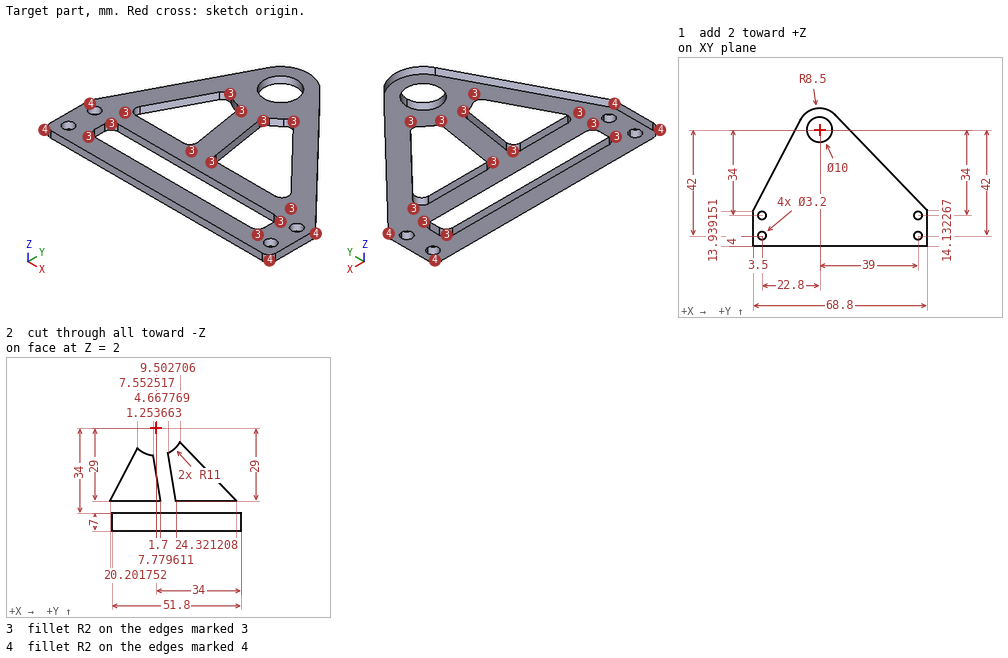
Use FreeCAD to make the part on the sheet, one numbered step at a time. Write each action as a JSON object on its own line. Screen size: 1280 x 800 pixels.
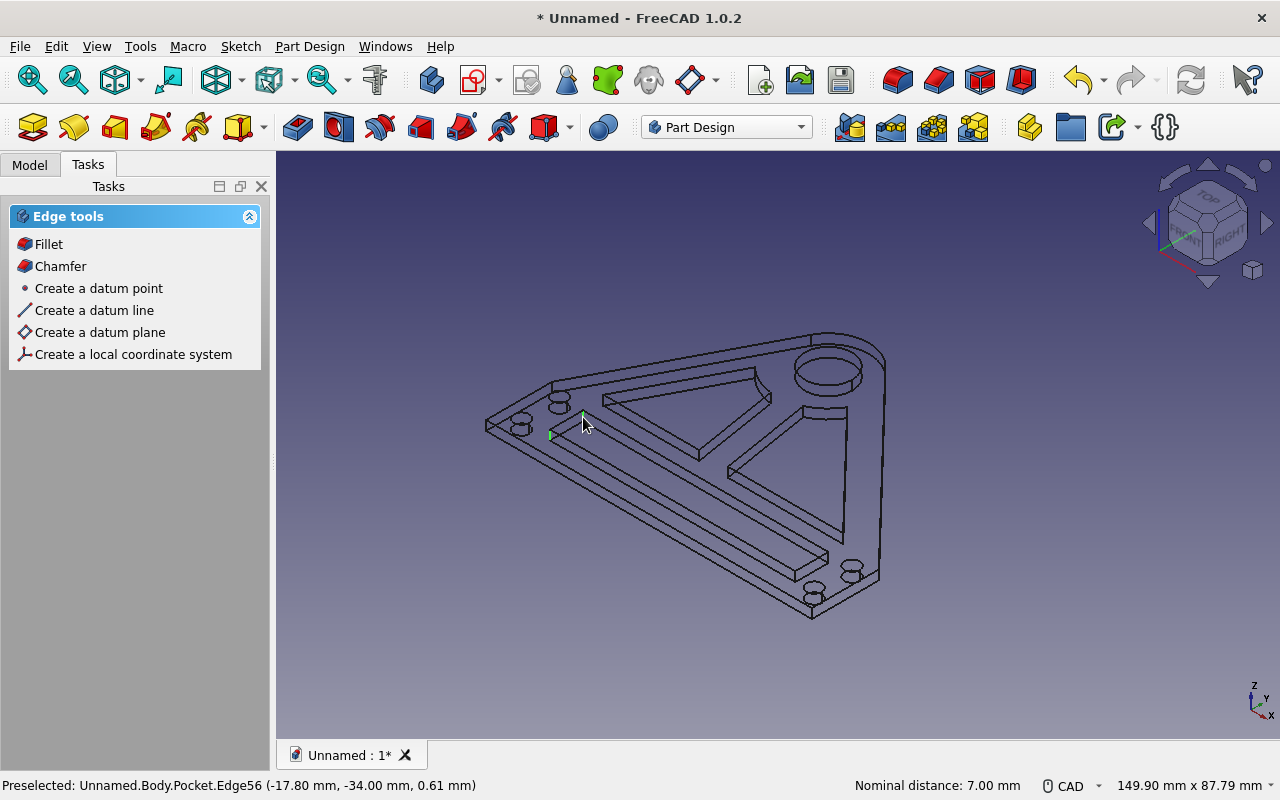
{"action": "left_click", "coordinate": [828, 559], "text": "ctrl"}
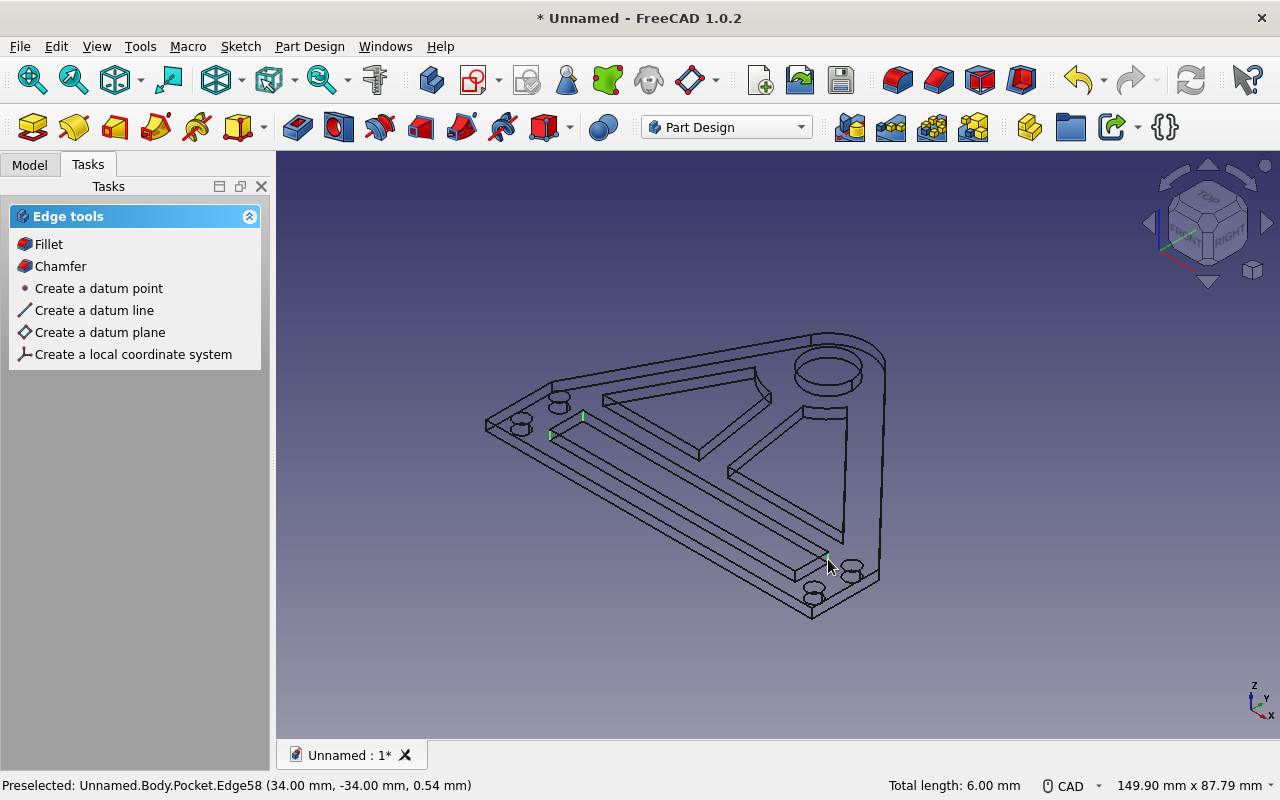
{"action": "left_click", "coordinate": [795, 577], "text": "ctrl"}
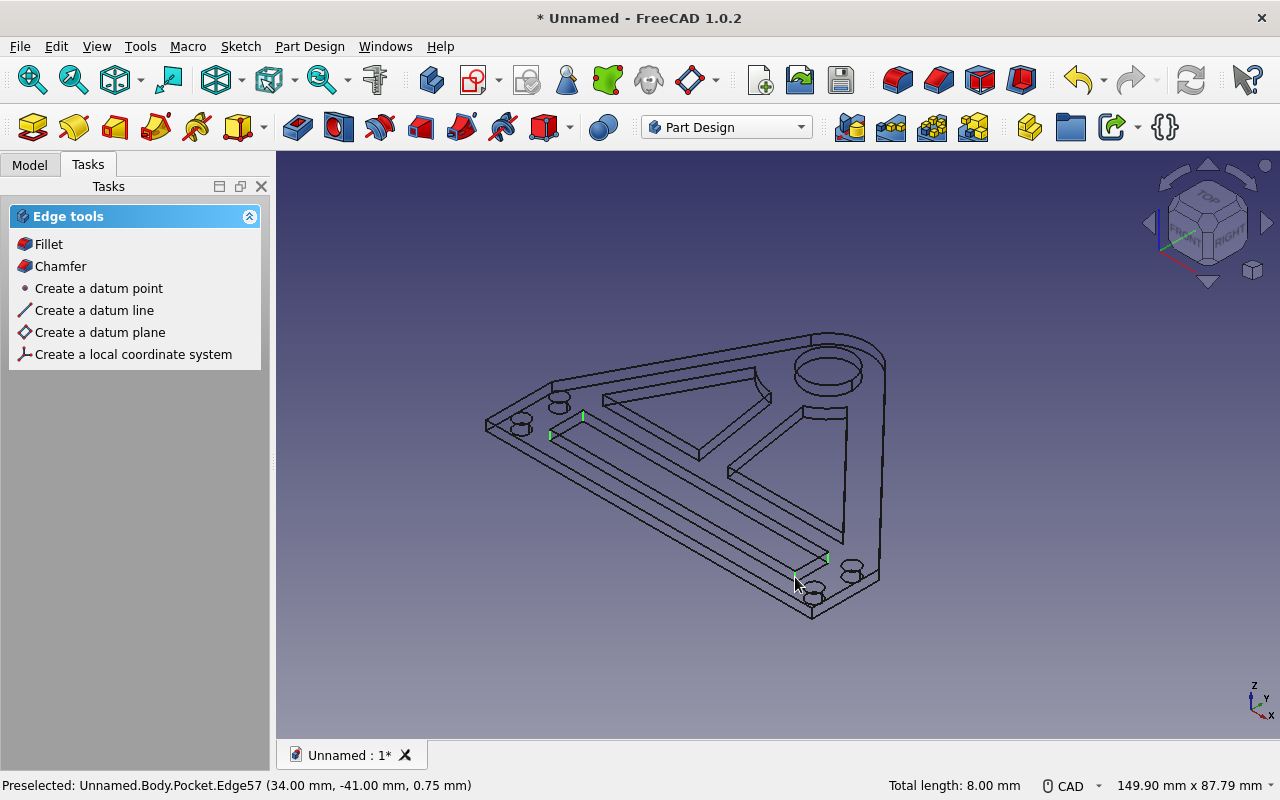
{"action": "left_click", "coordinate": [843, 539], "text": "ctrl"}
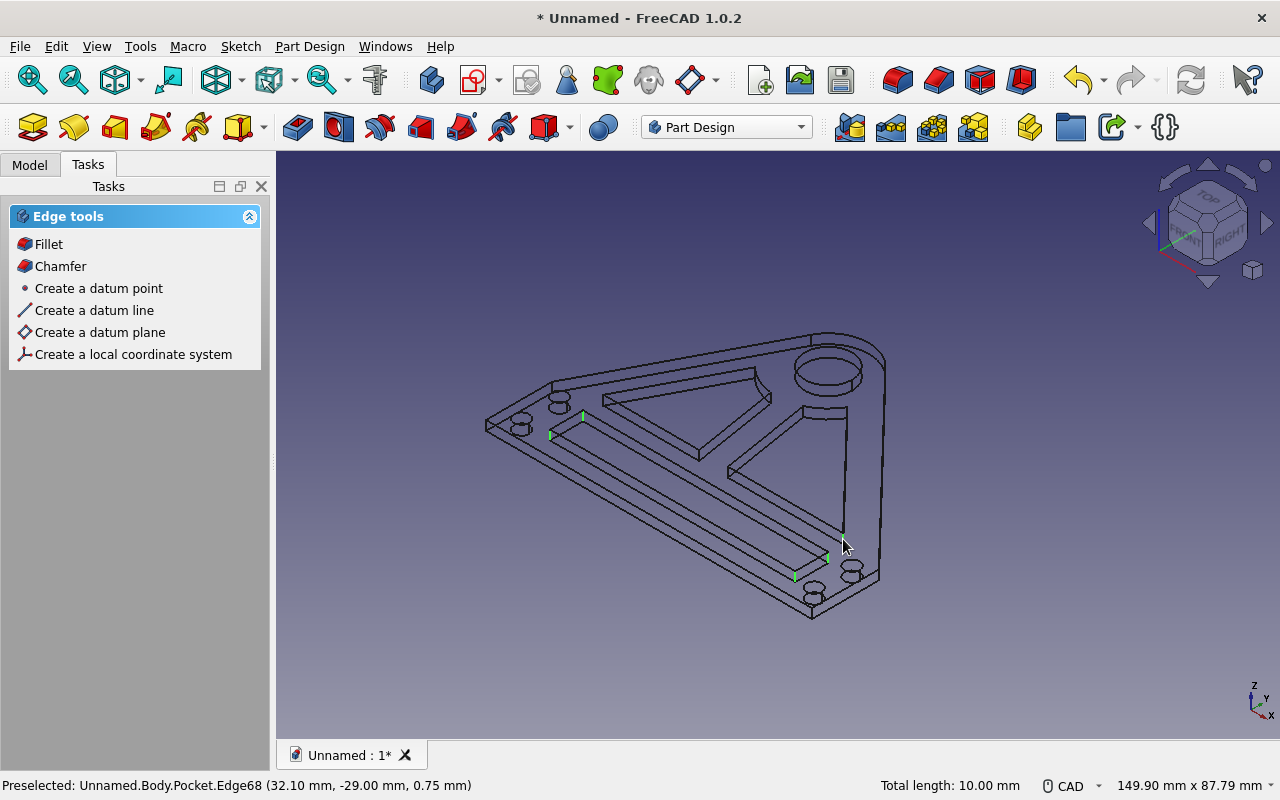
{"action": "left_click", "coordinate": [728, 474], "text": "ctrl"}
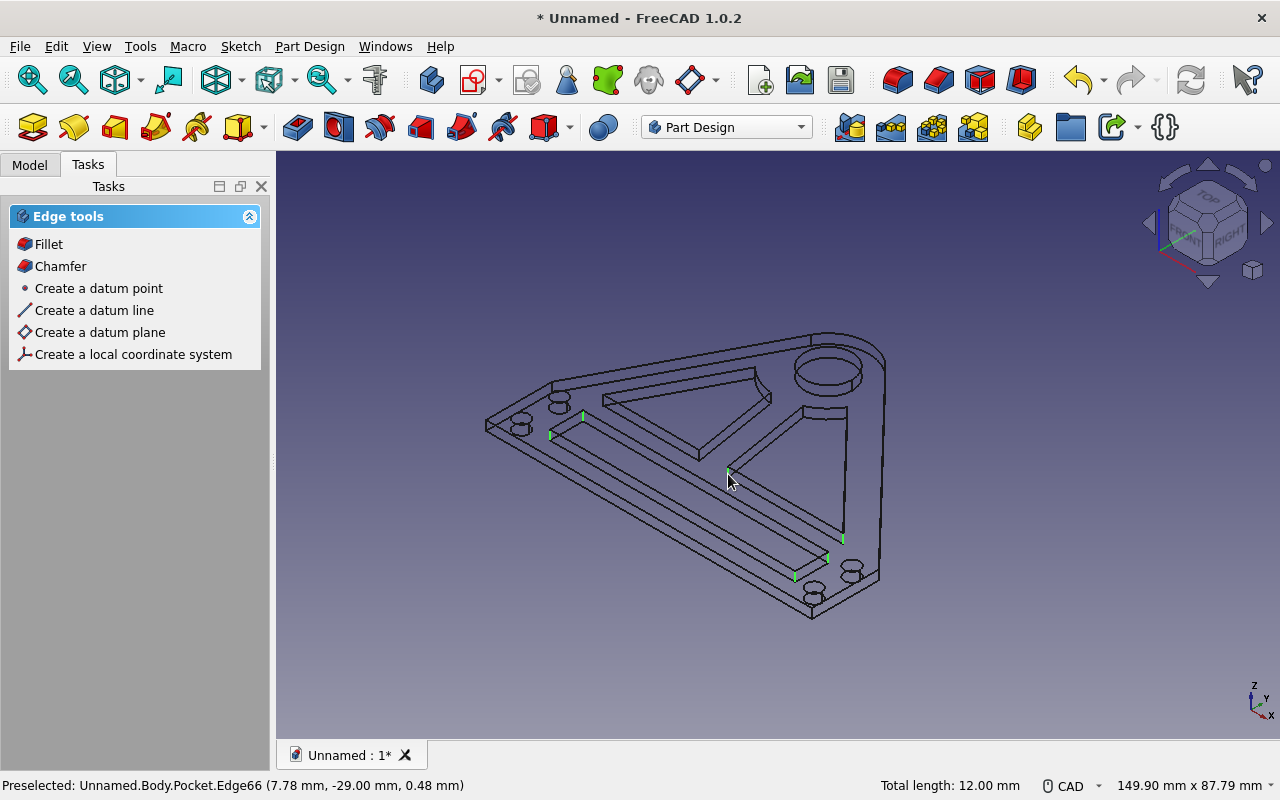
{"action": "left_click", "coordinate": [771, 400], "text": "ctrl"}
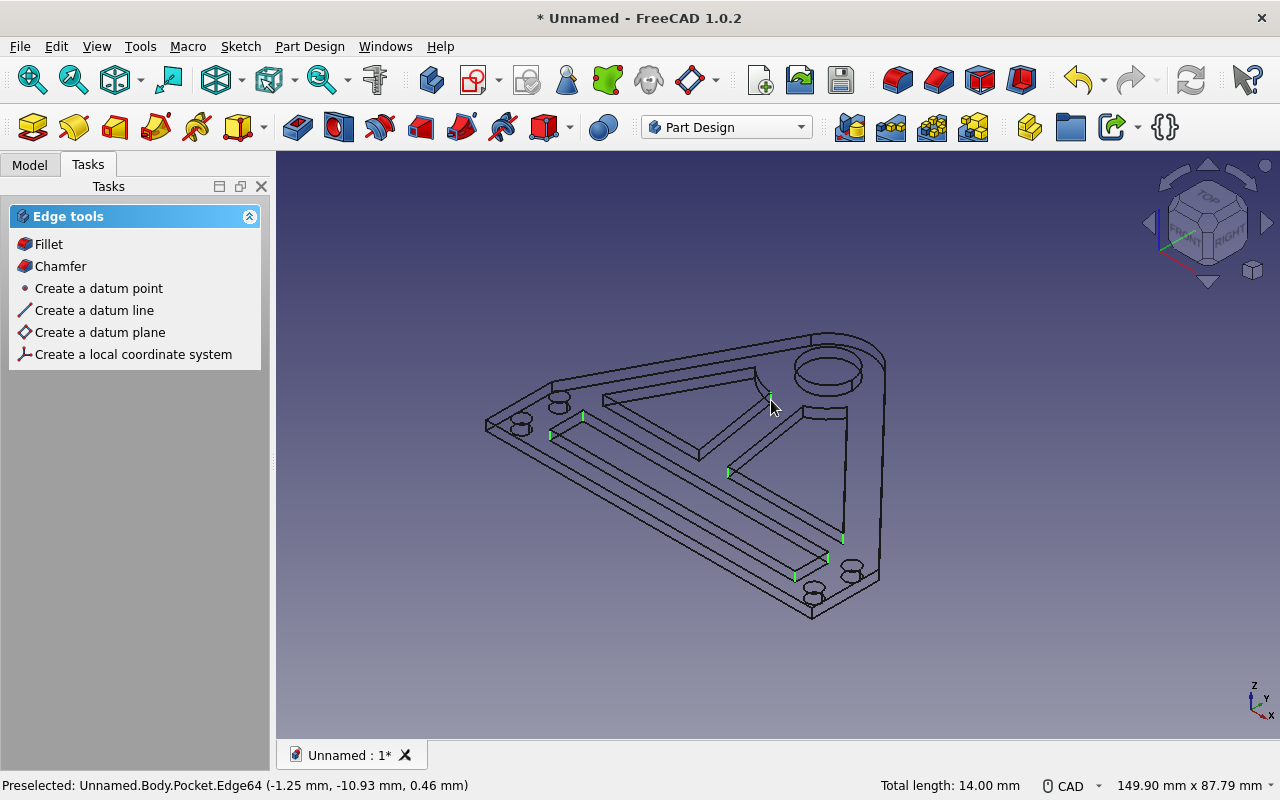
{"action": "left_click", "coordinate": [699, 455], "text": "ctrl"}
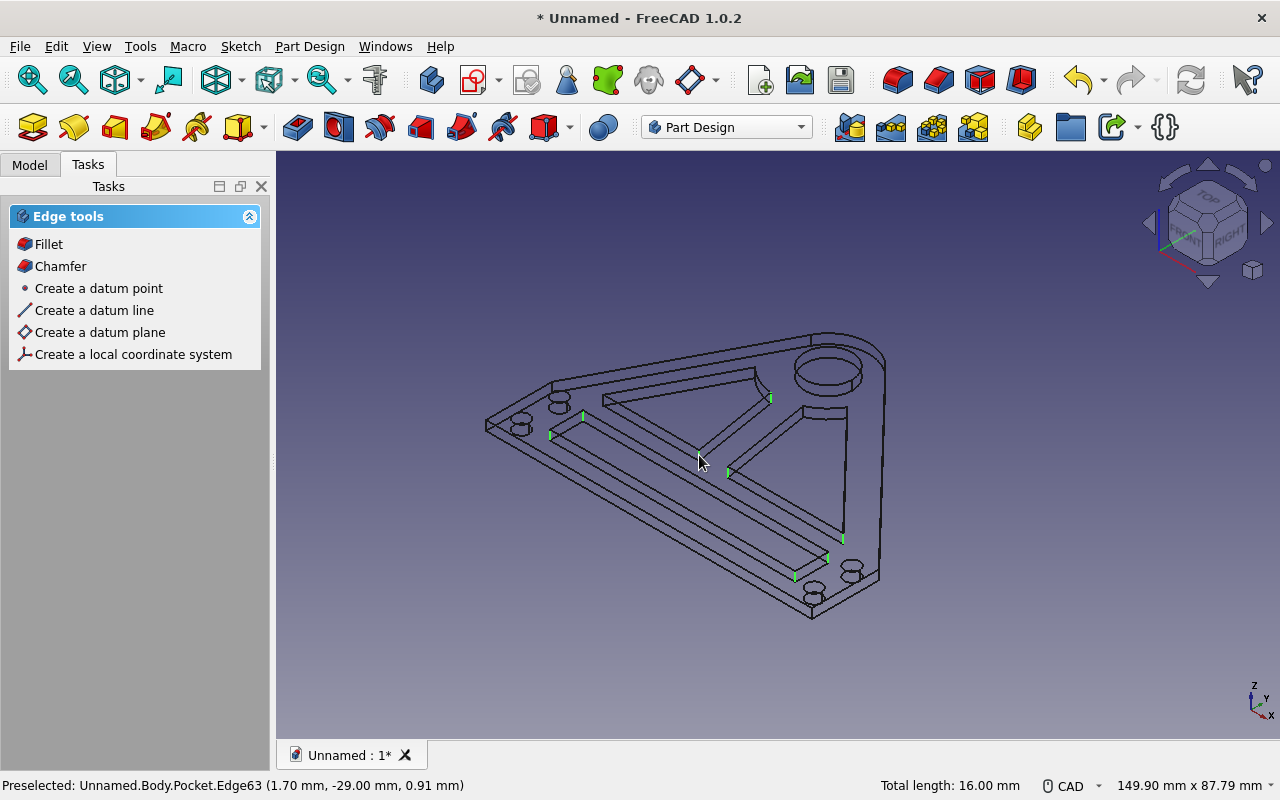
{"action": "left_click", "coordinate": [603, 401], "text": "ctrl"}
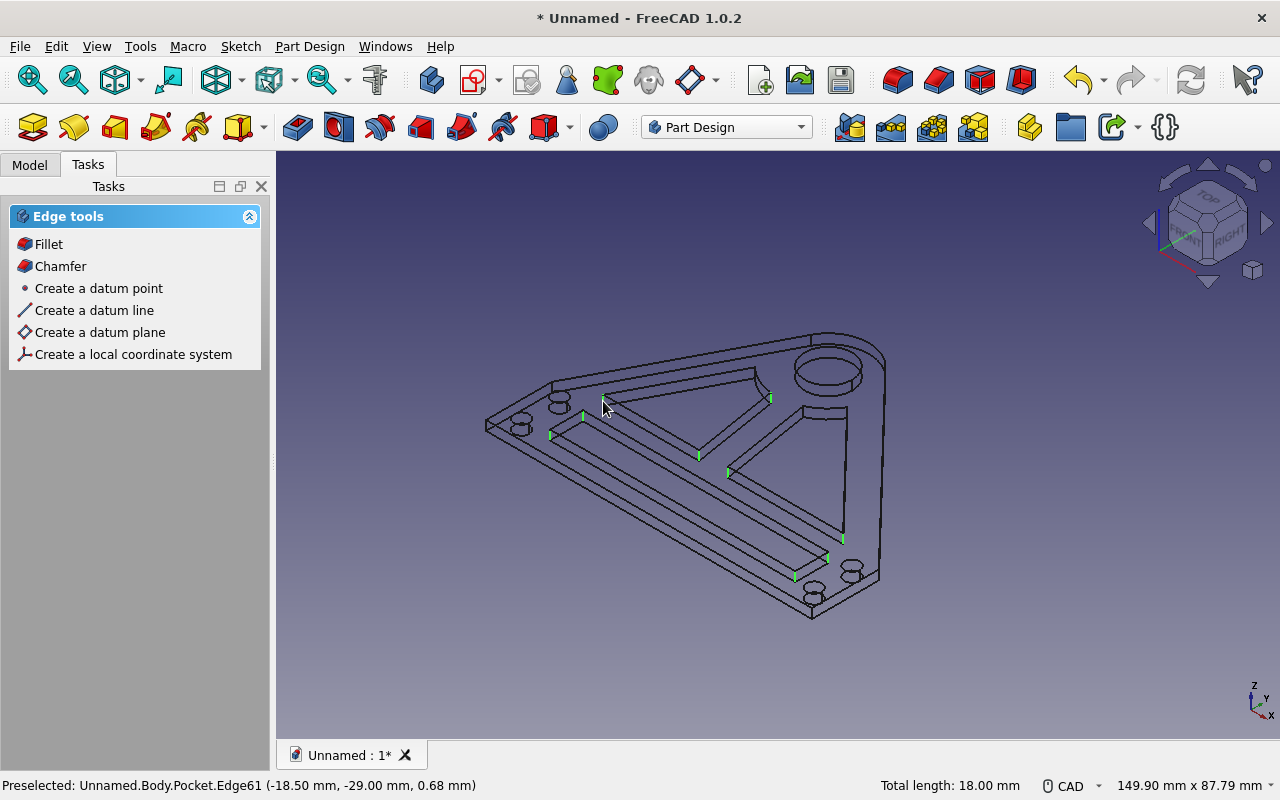
{"action": "scroll", "coordinate": [803, 411], "scroll_direction": "up", "scroll_amount": 6}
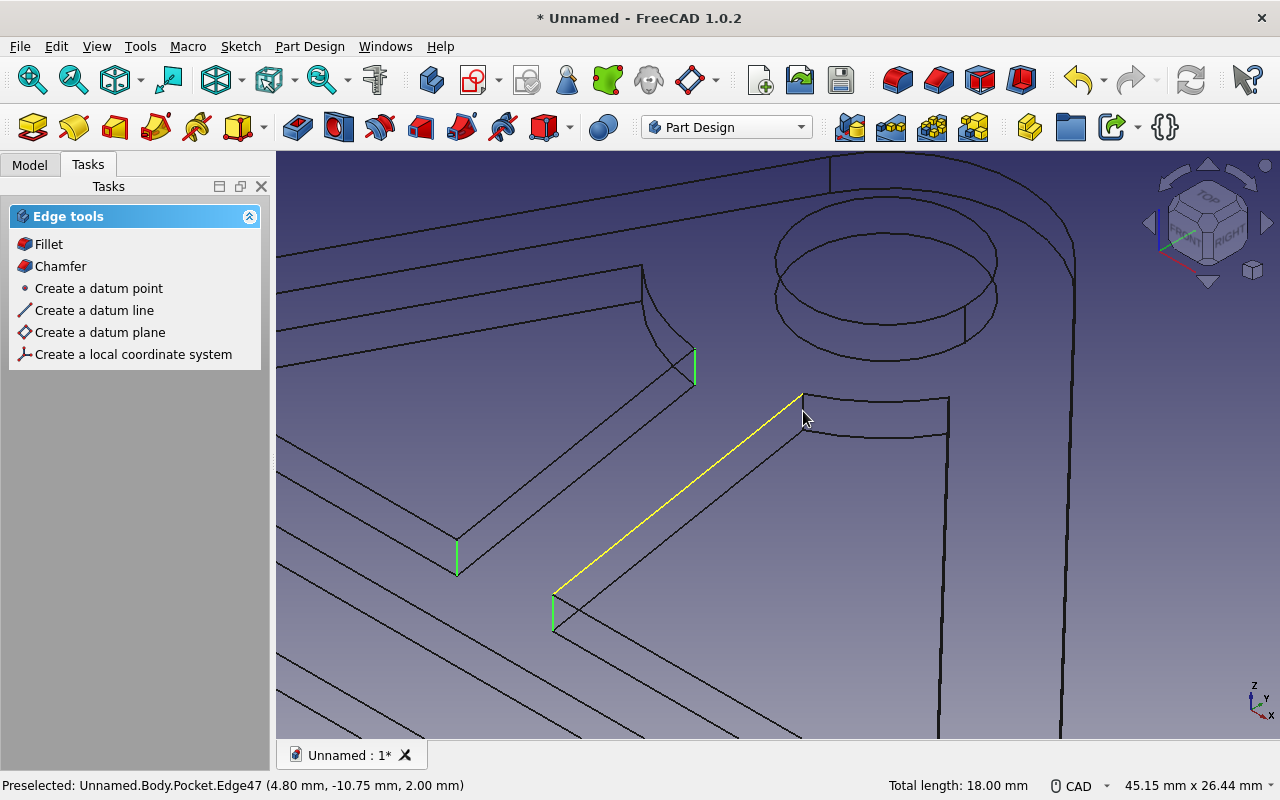
{"action": "left_click", "coordinate": [803, 411], "text": "ctrl"}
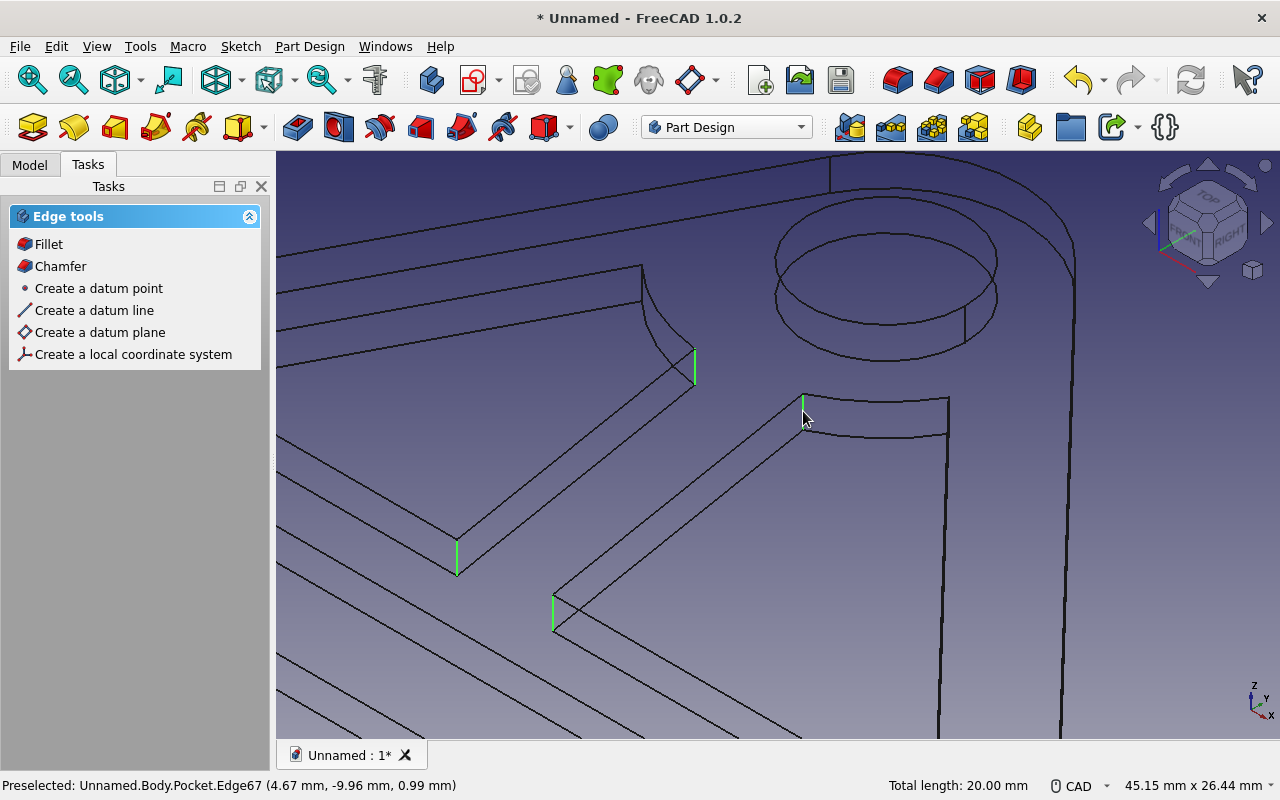
{"action": "left_click", "coordinate": [642, 293], "text": "ctrl"}